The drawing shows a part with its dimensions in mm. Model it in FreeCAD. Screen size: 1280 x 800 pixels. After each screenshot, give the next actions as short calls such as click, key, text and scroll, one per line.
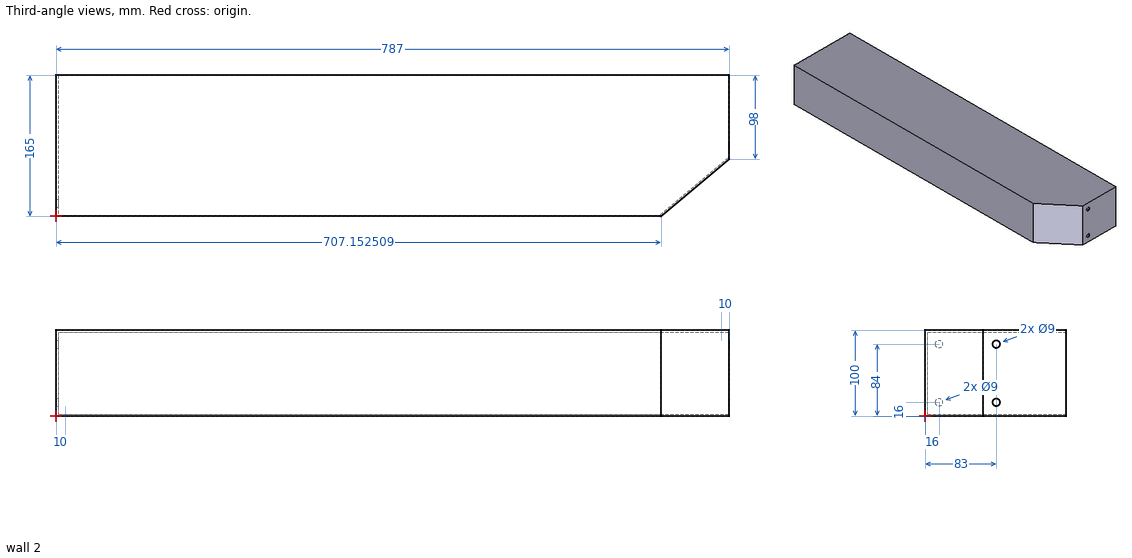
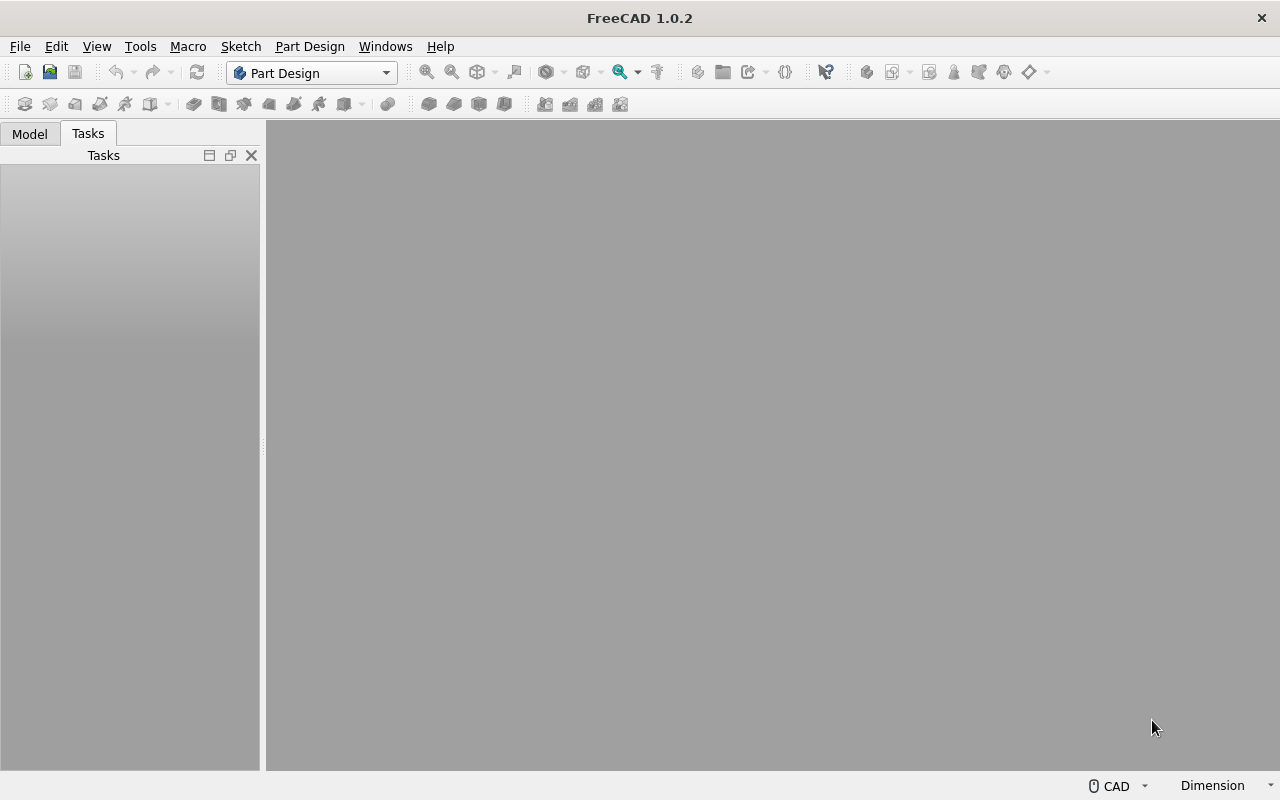
click(25, 72)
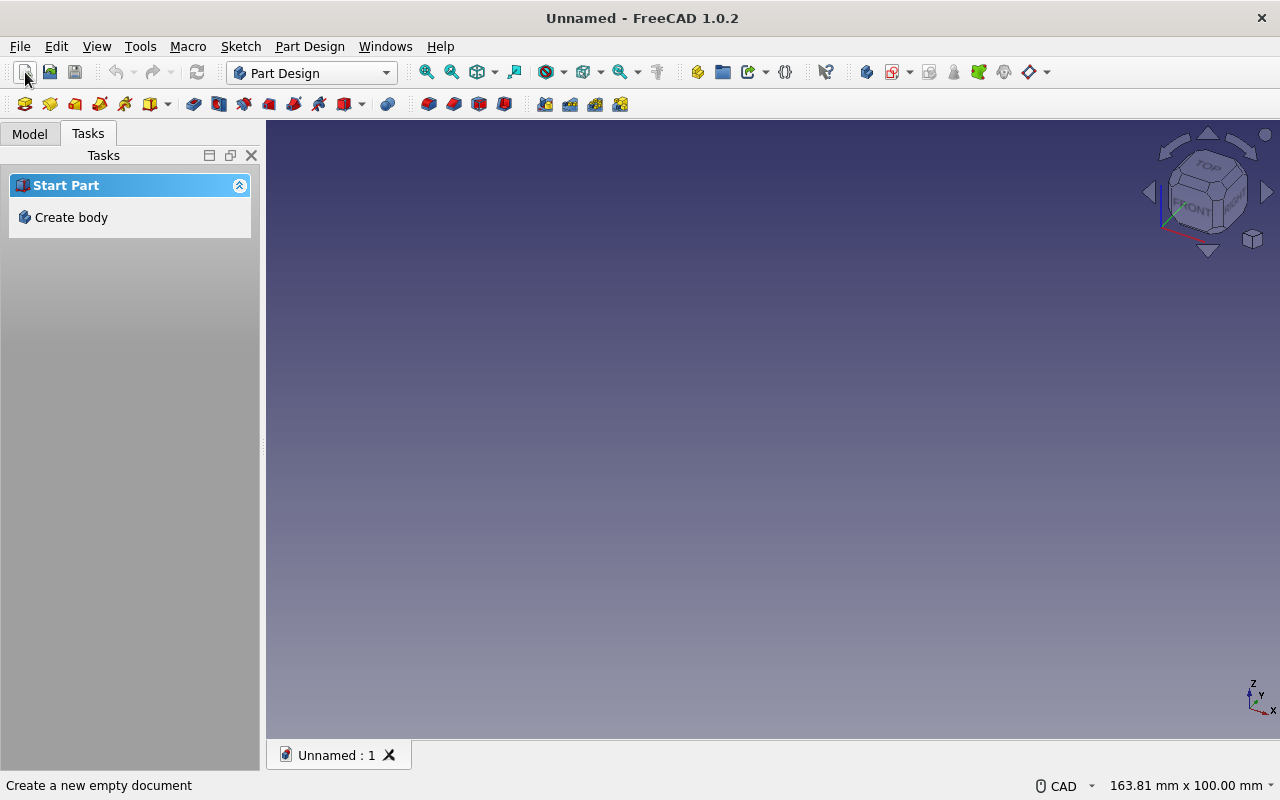
click(892, 72)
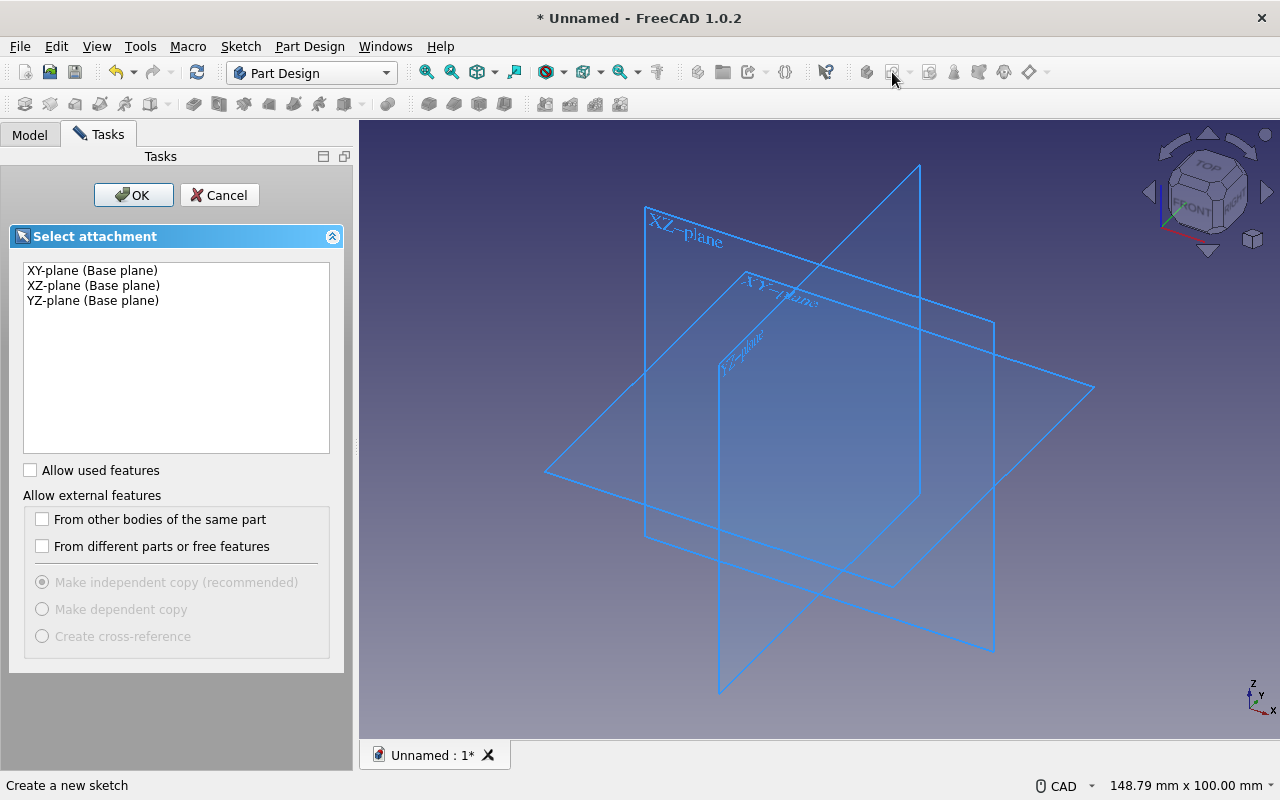
click(84, 270)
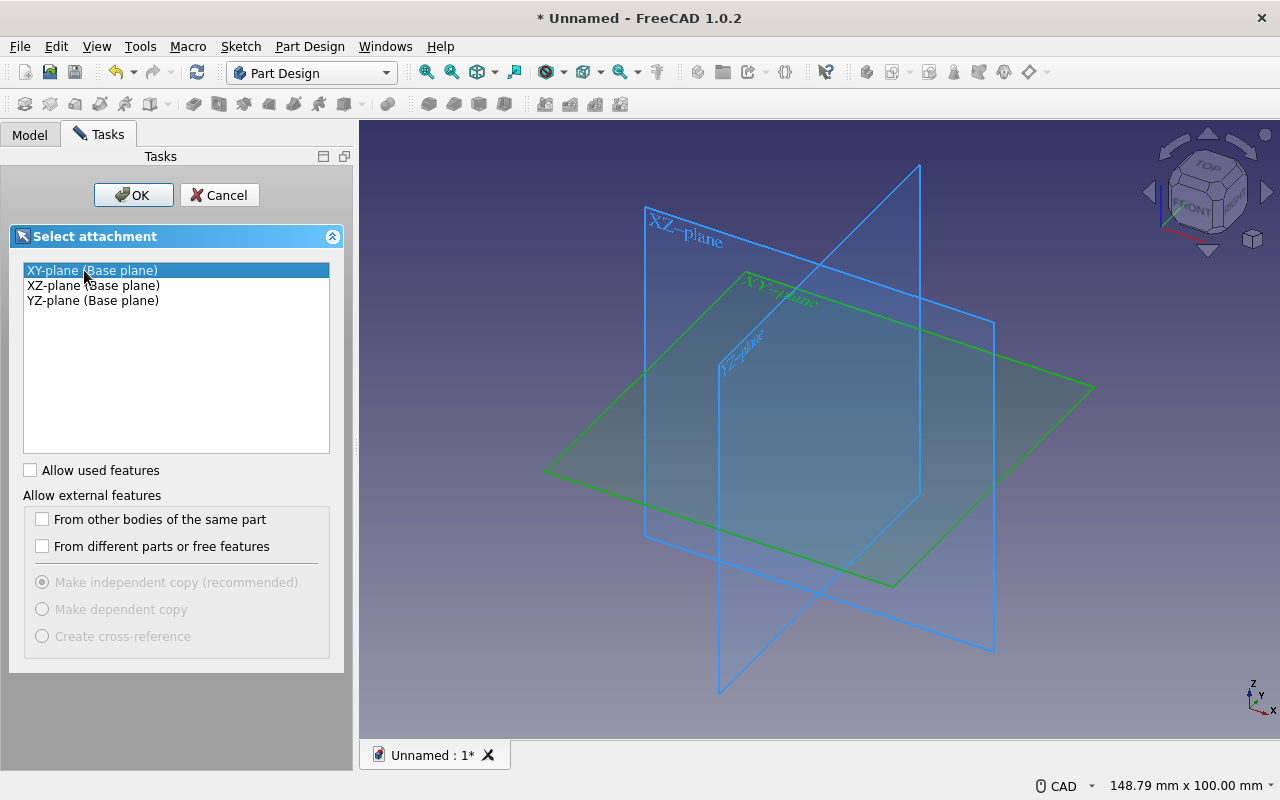
click(134, 195)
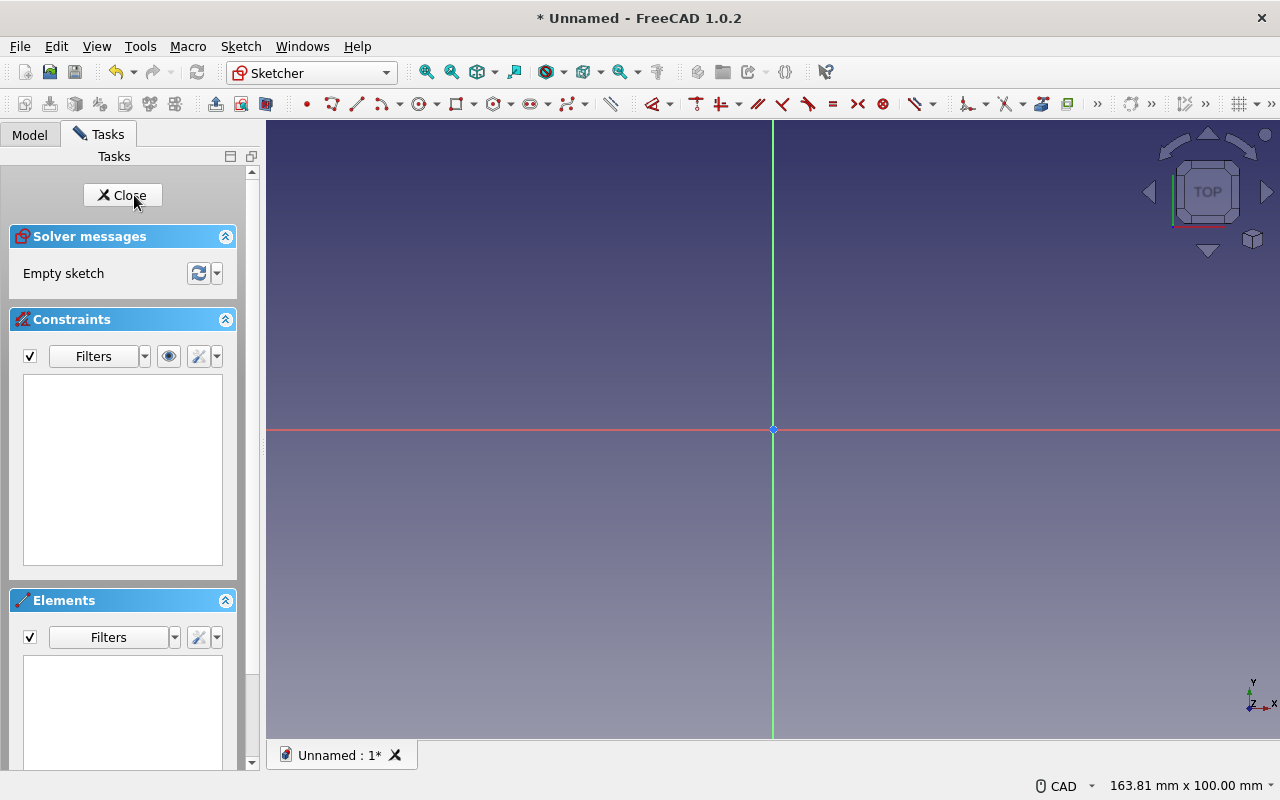
scroll(392, 493, down, 11)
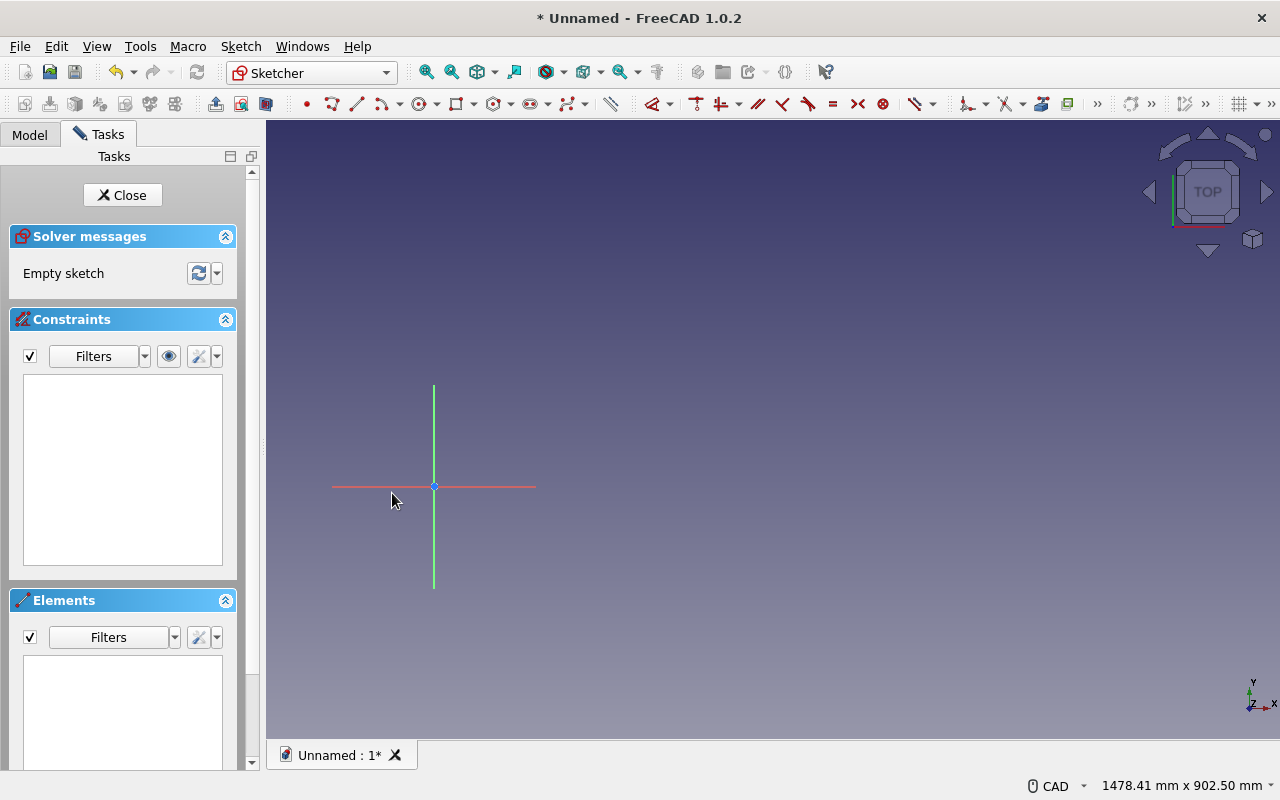
click(332, 104)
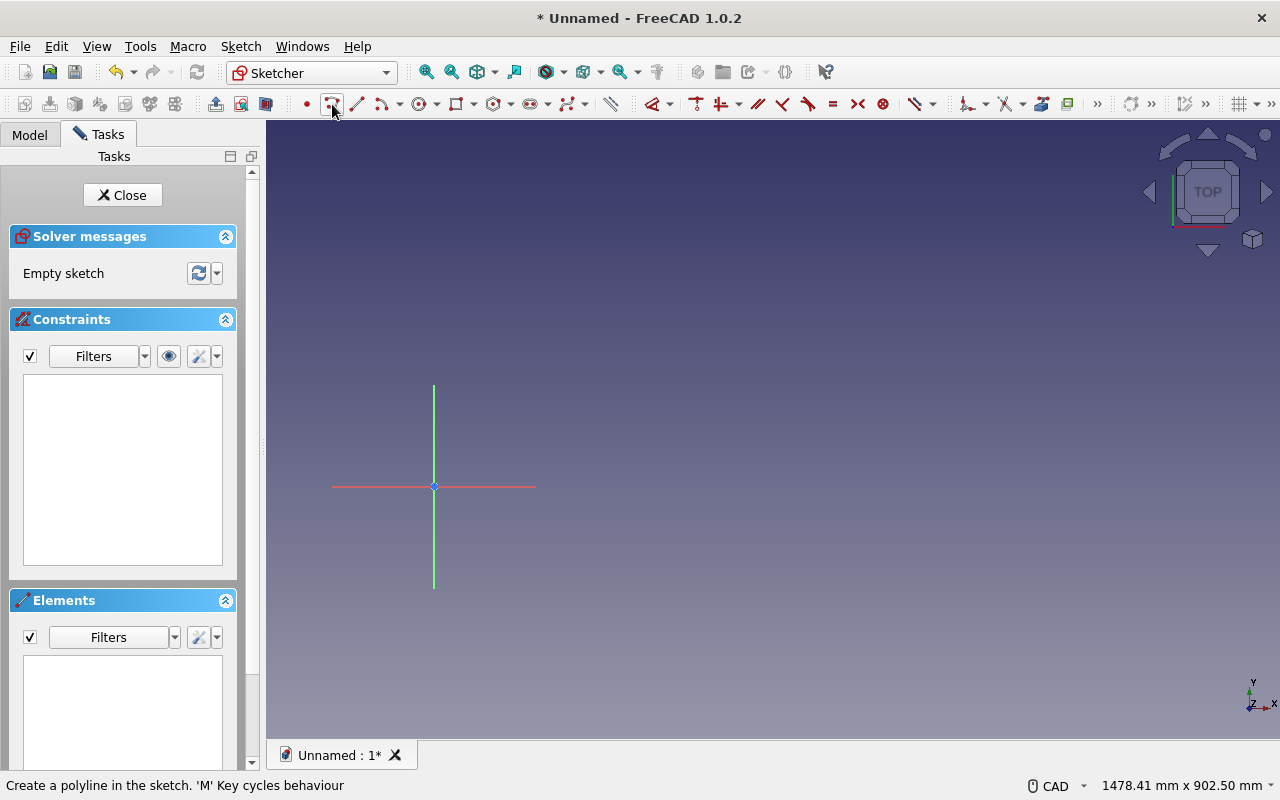
click(434, 487)
click(919, 478)
click(974, 441)
click(974, 373)
click(443, 373)
click(434, 487)
key(Escape)
key(Escape)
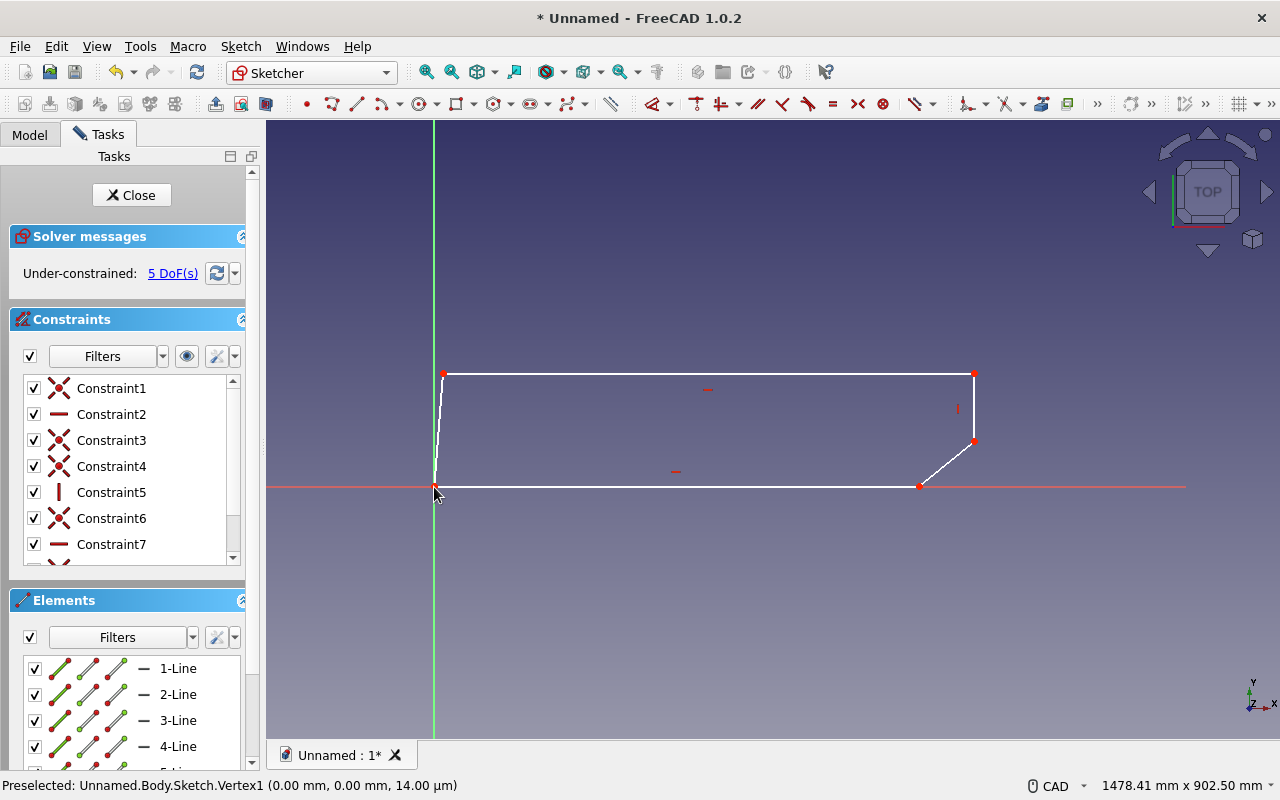
click(437, 453)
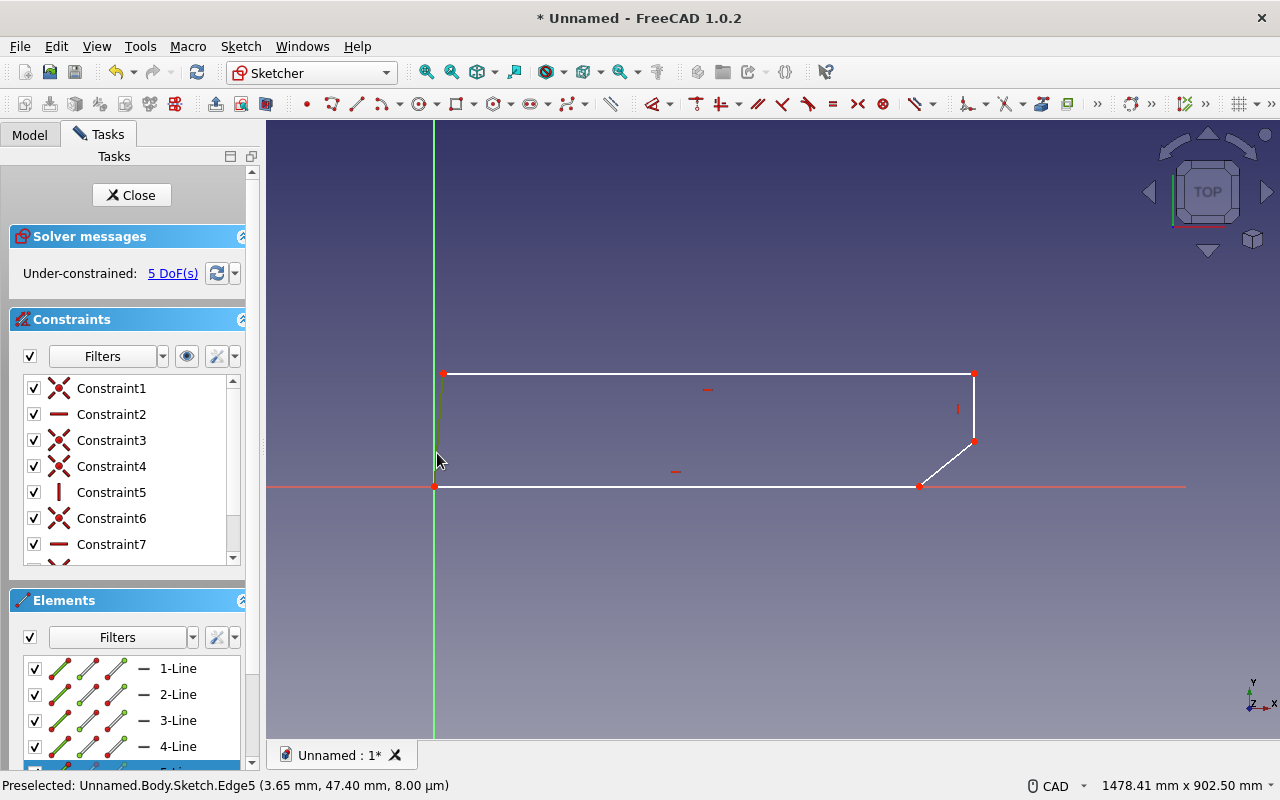
click(738, 104)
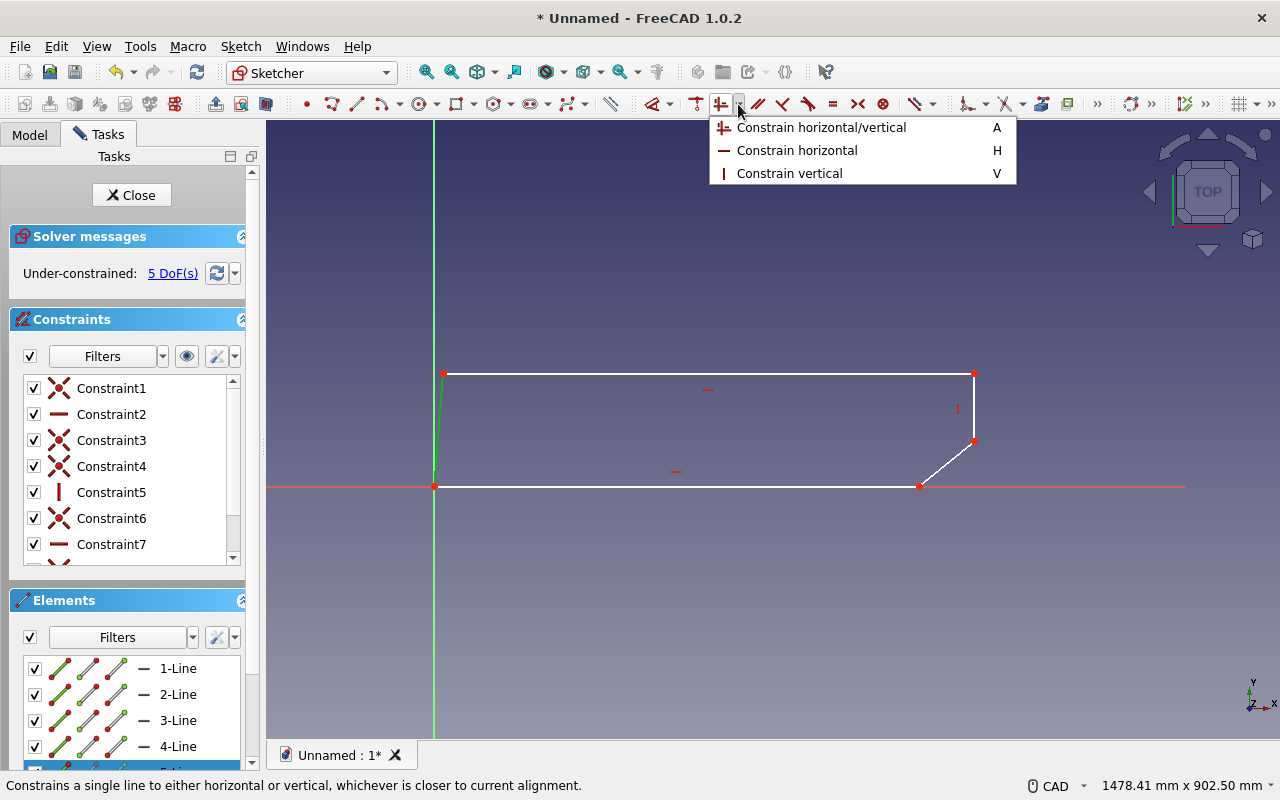
click(863, 174)